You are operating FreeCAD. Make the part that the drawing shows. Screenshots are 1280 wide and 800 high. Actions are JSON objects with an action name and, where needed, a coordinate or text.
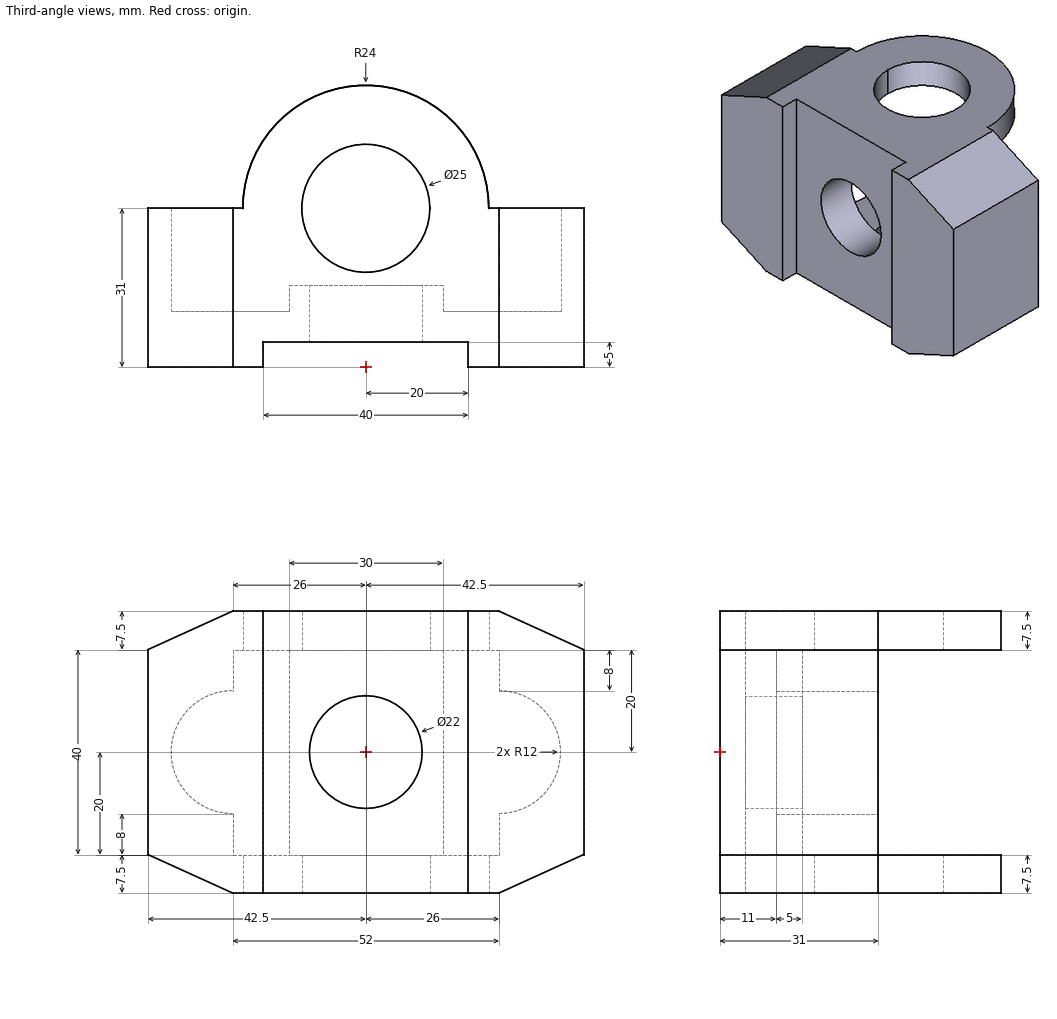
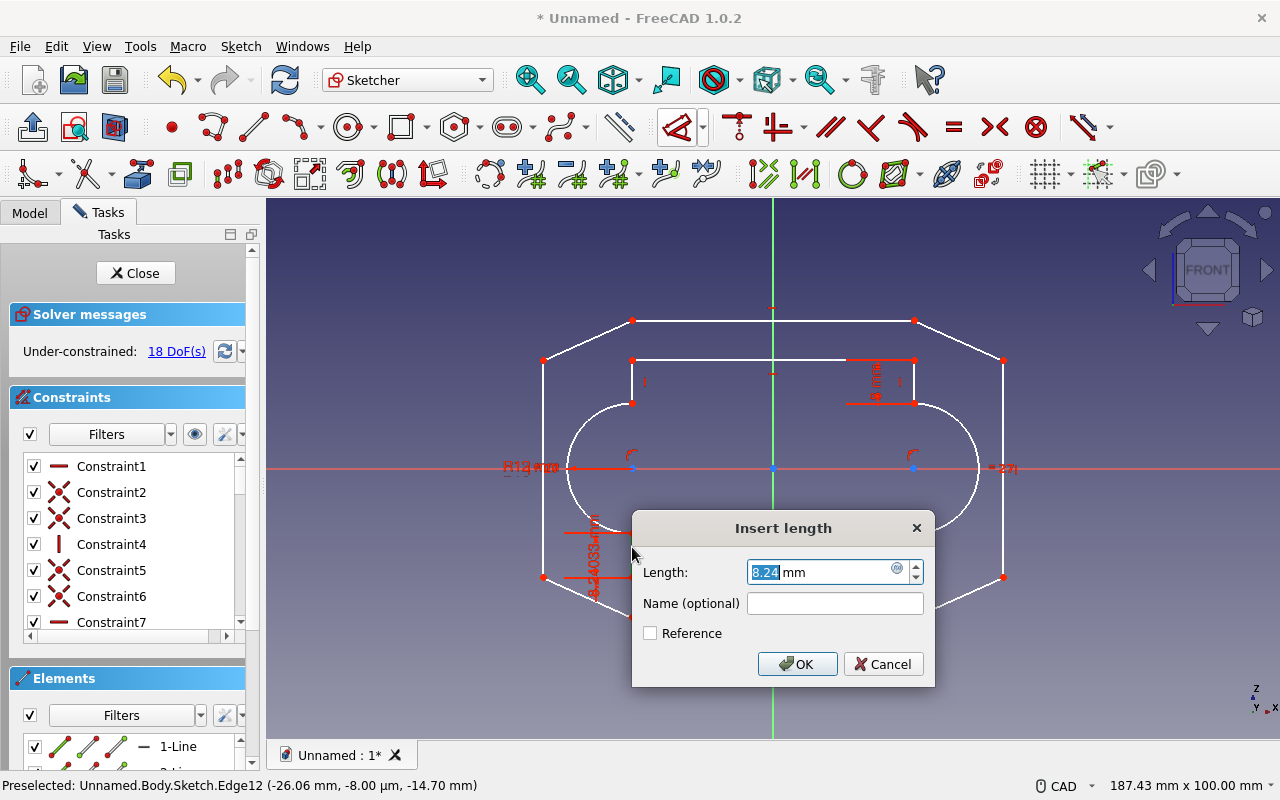
{"action": "type", "text": "8"}
{"action": "key", "text": "Return"}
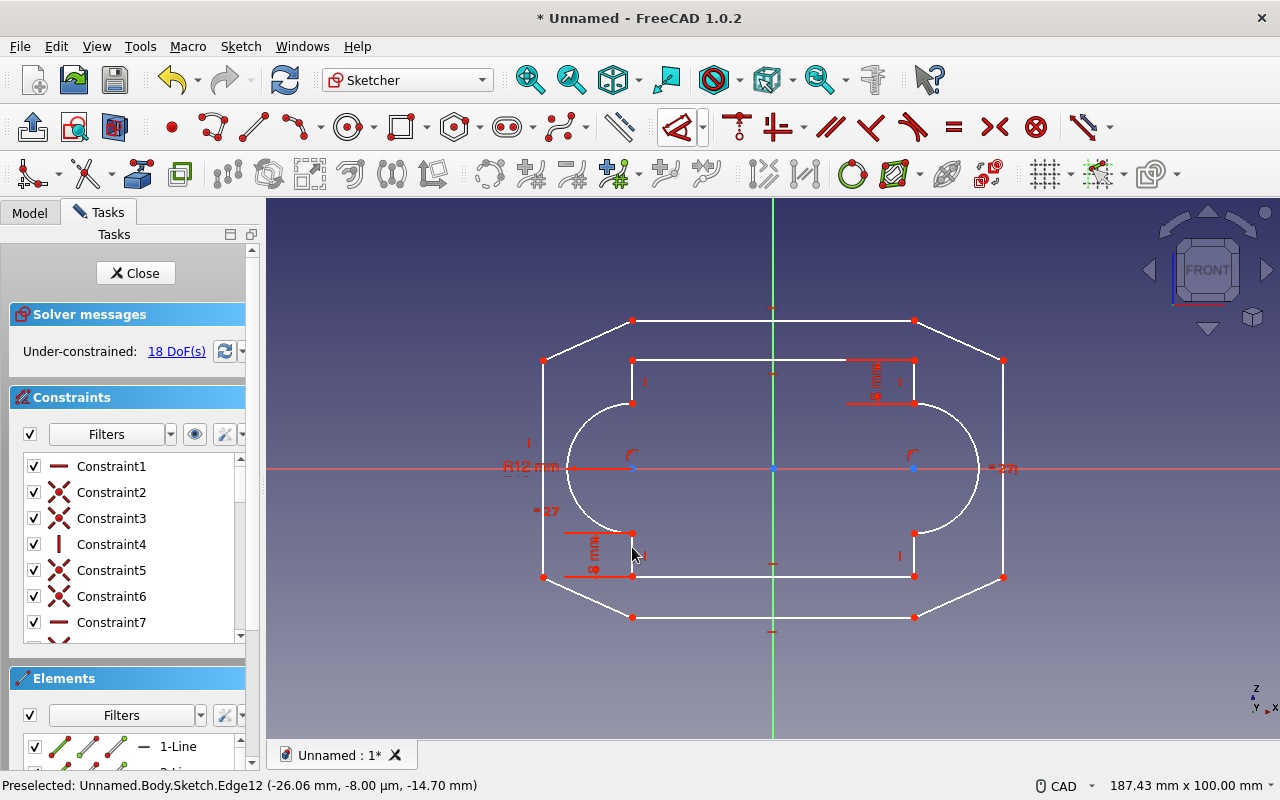
{"action": "left_click", "coordinate": [829, 618]}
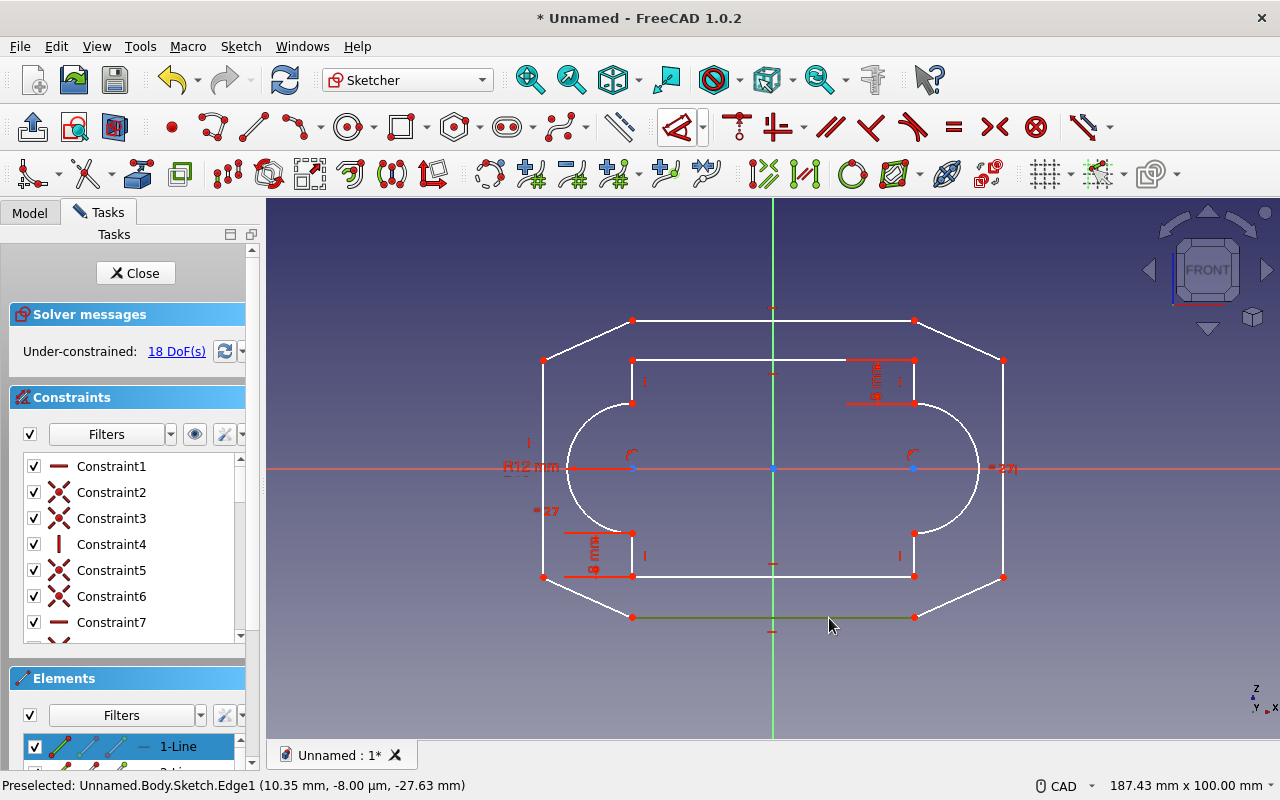
{"action": "key", "text": "l"}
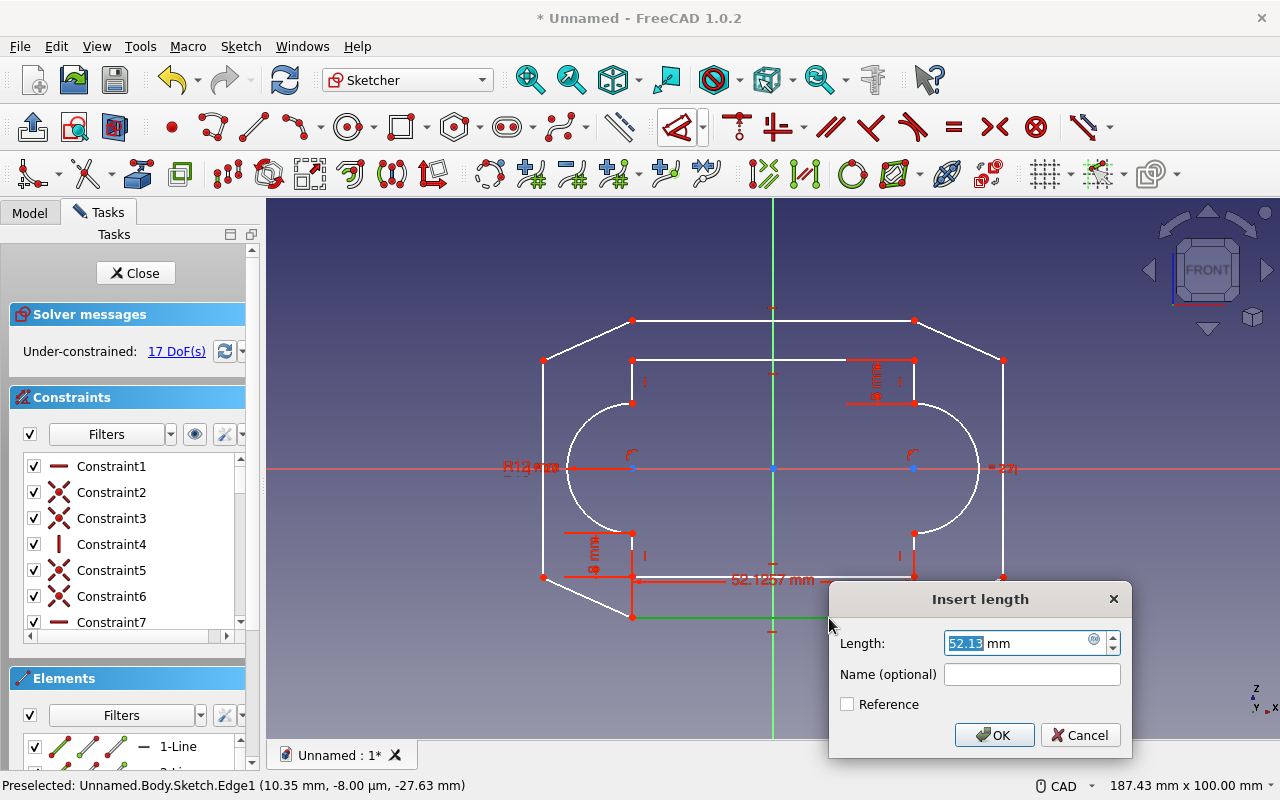
{"action": "type", "text": "52"}
{"action": "key", "text": "Return"}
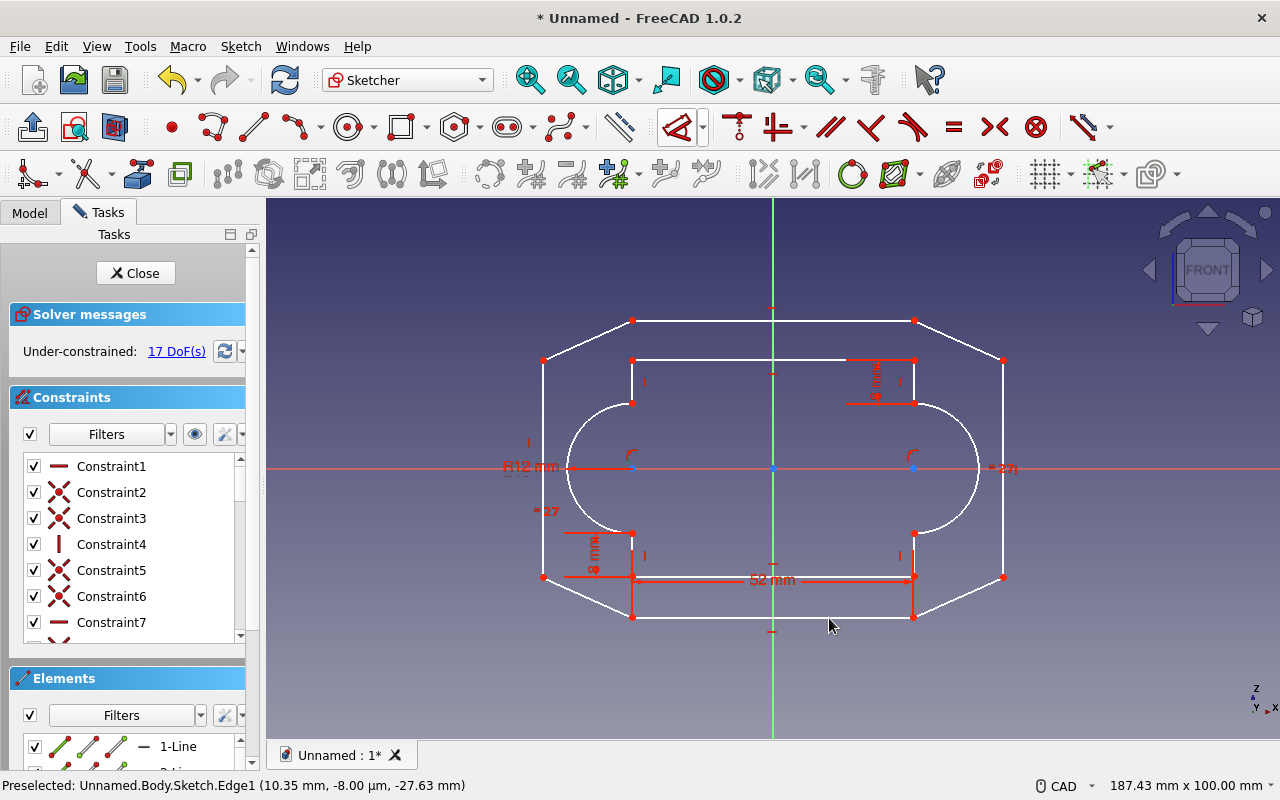
{"action": "left_click", "coordinate": [543, 426]}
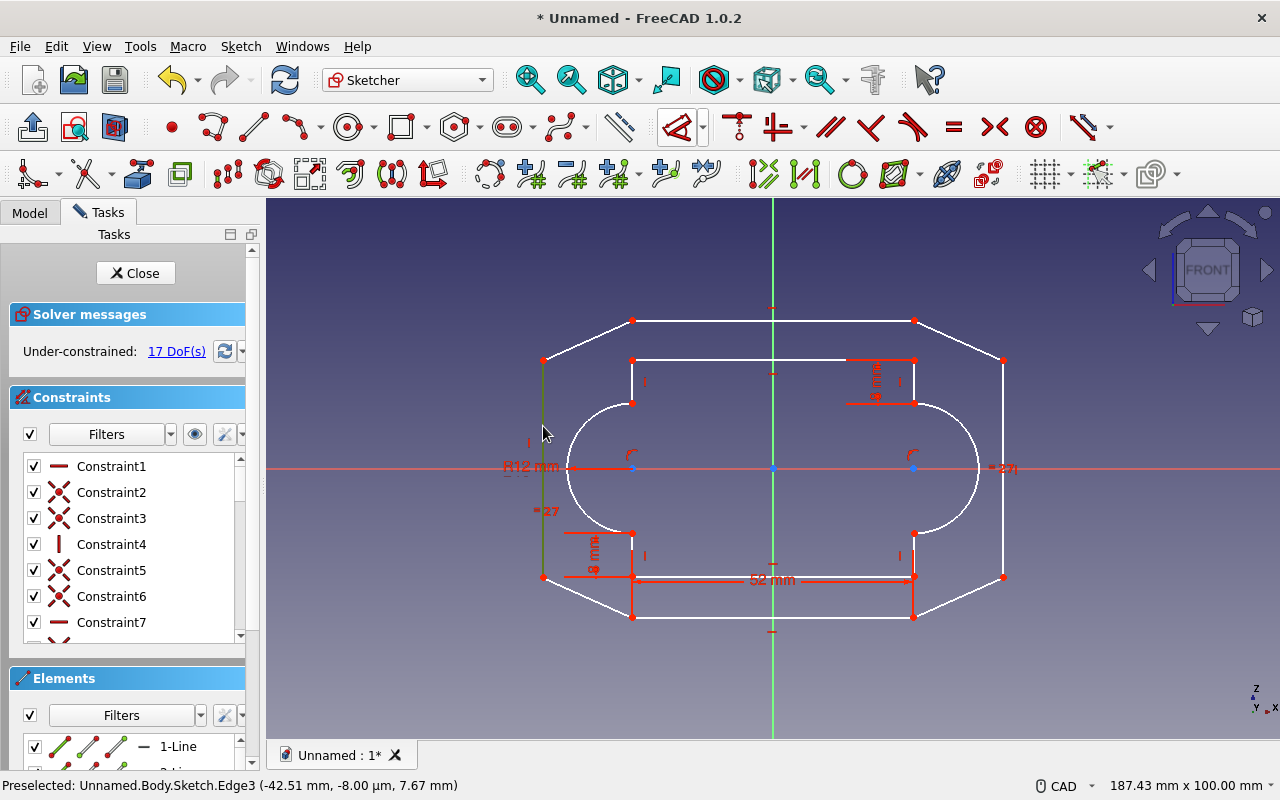
{"action": "left_click", "coordinate": [702, 128]}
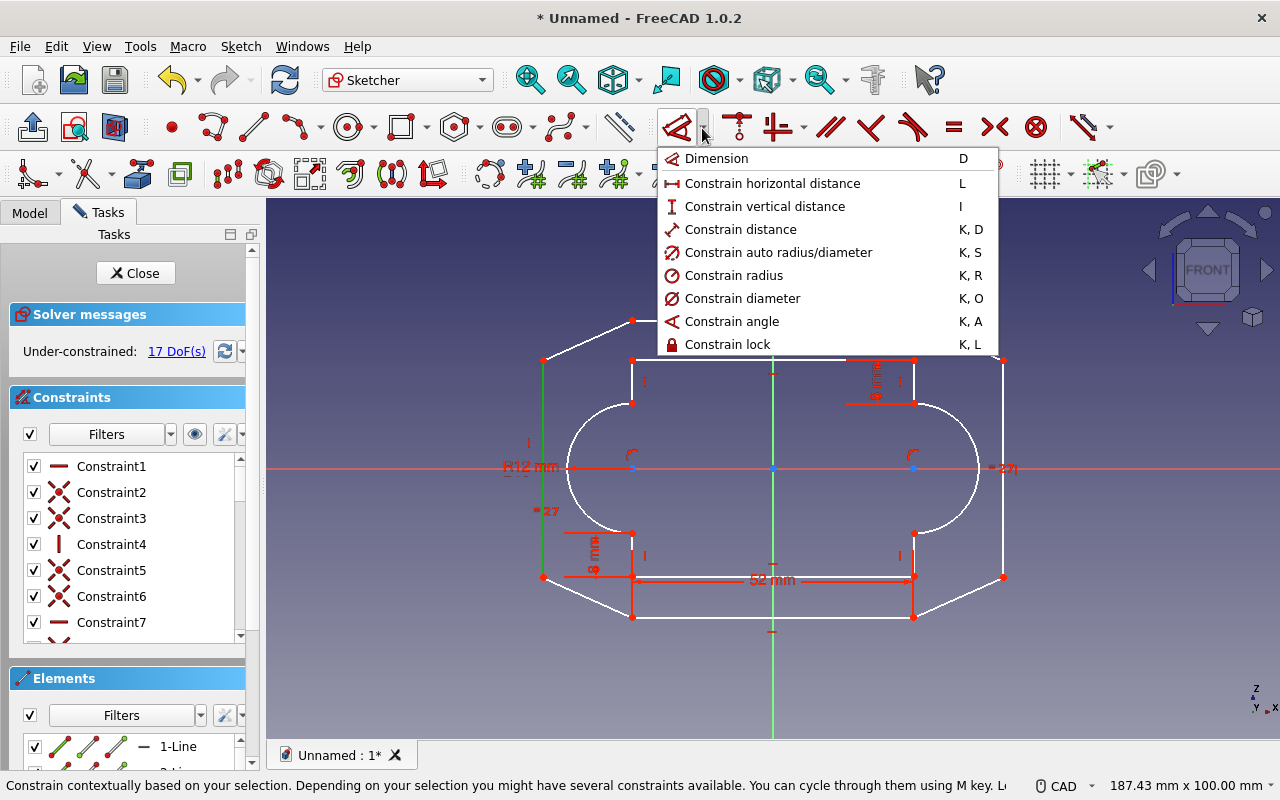
{"action": "left_click", "coordinate": [828, 206]}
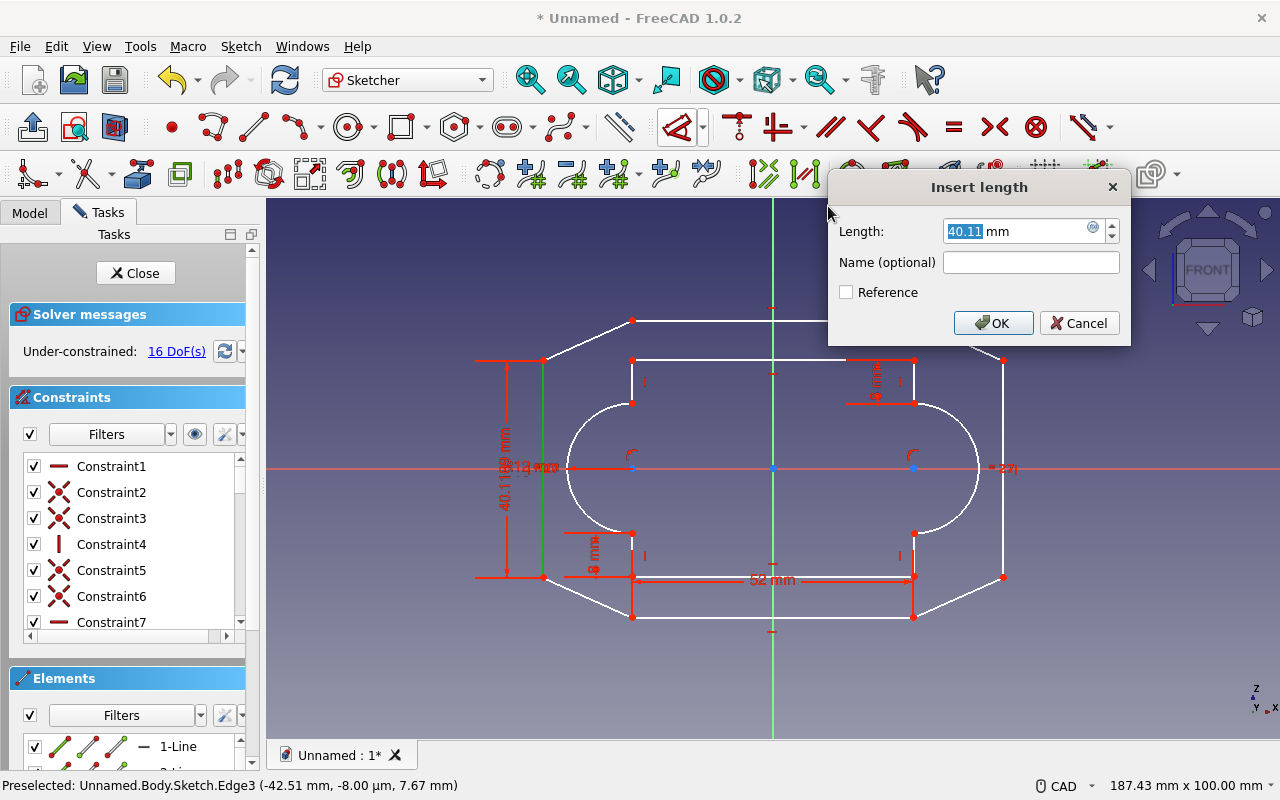
{"action": "type", "text": "40"}
{"action": "key", "text": "Return"}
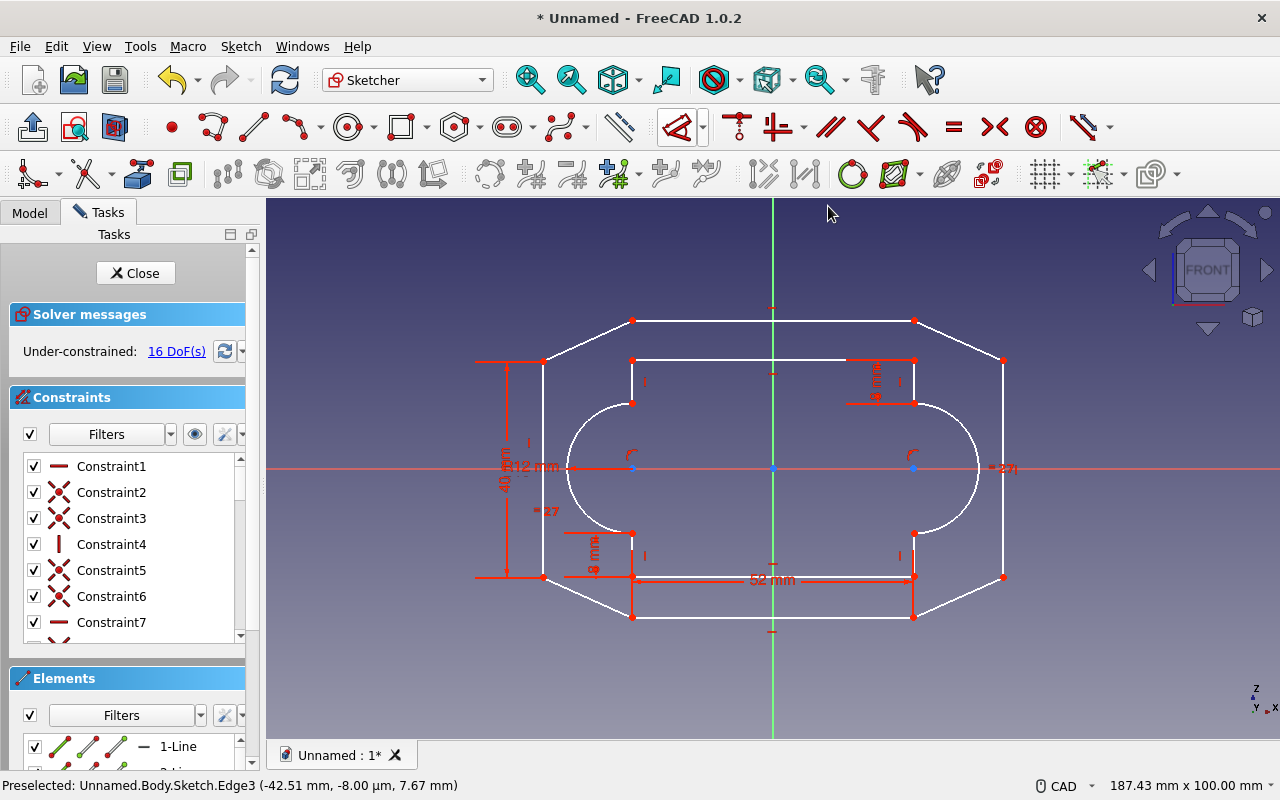
{"action": "left_click", "coordinate": [717, 321]}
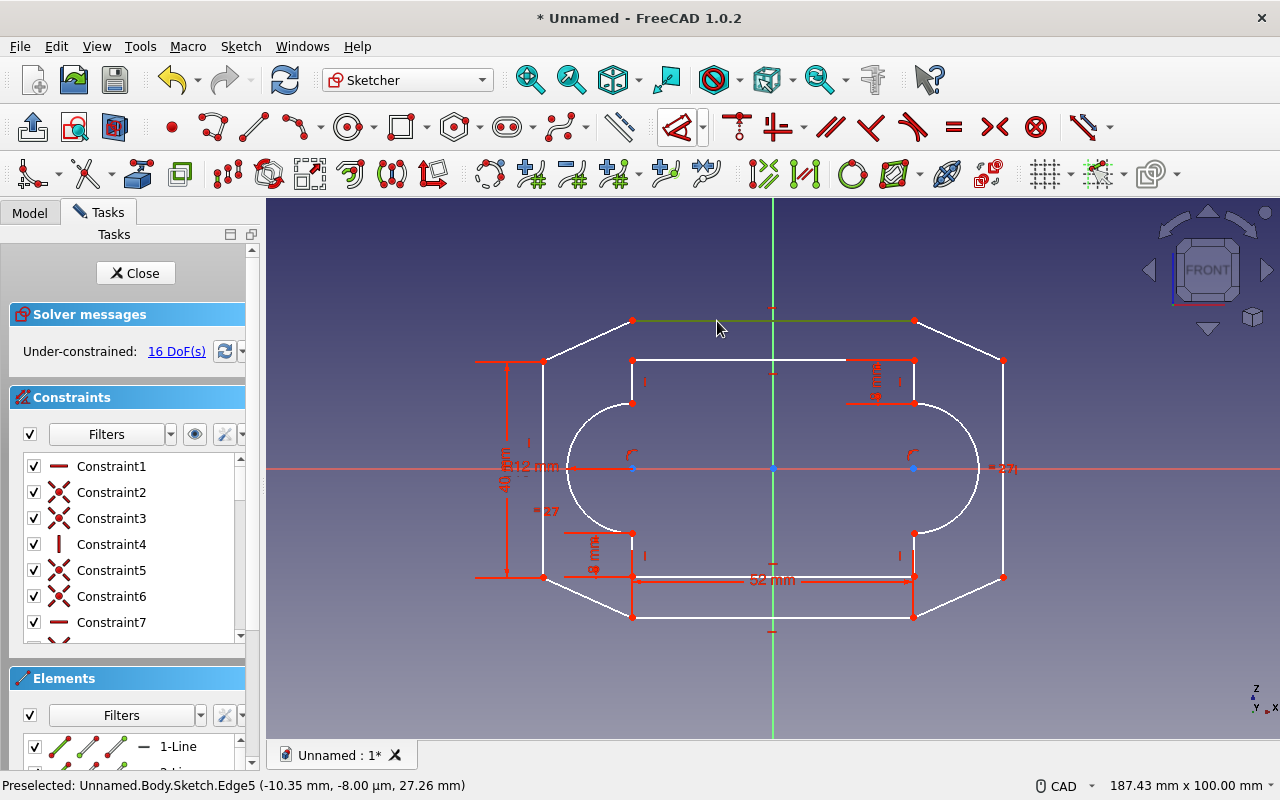
{"action": "key", "text": "l"}